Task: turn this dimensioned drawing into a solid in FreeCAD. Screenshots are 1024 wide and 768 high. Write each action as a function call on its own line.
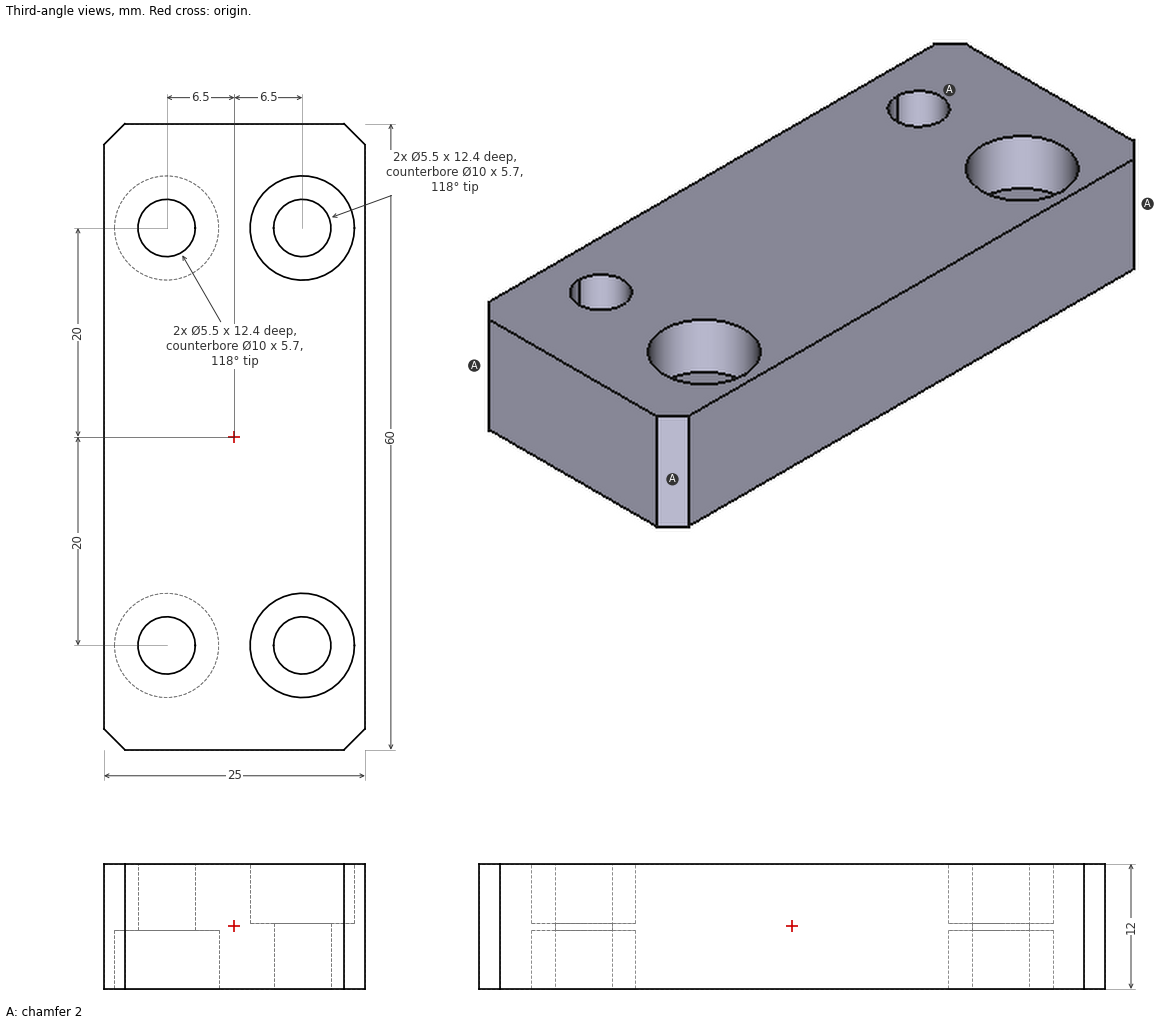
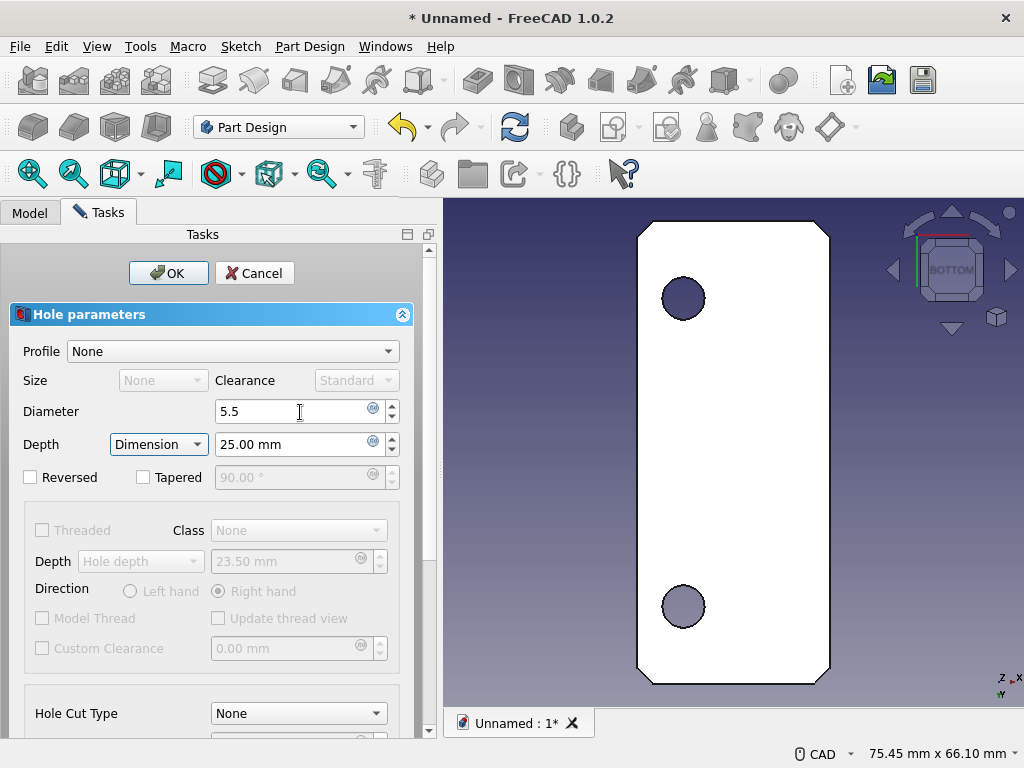
triple_click(300, 444)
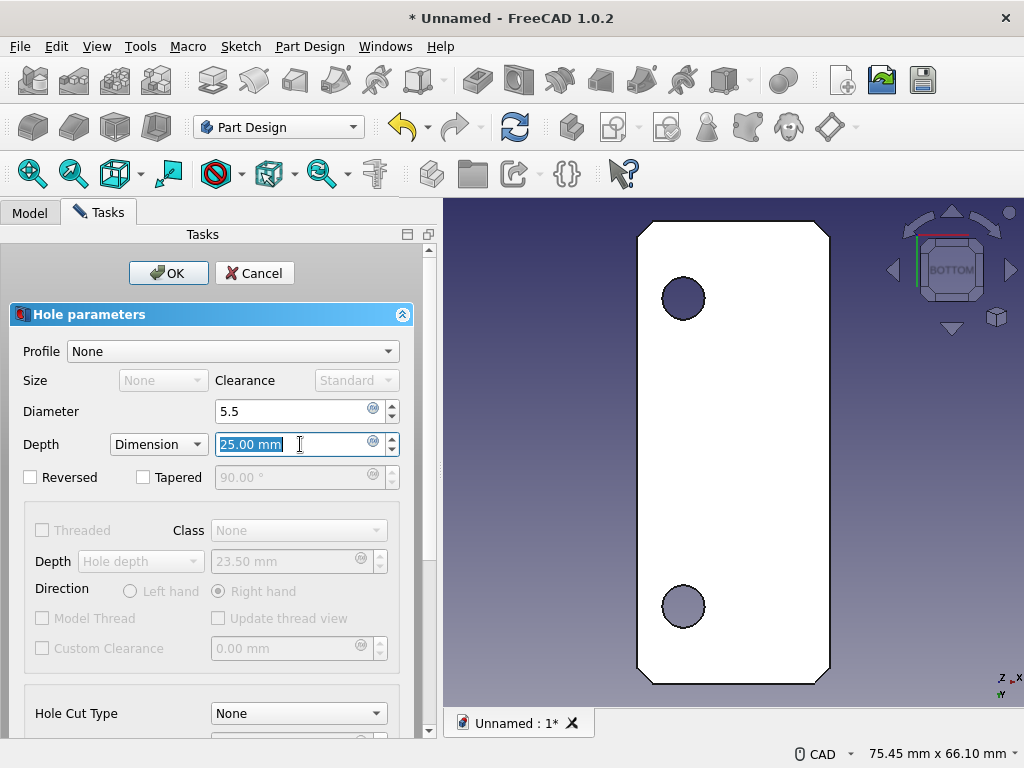
text(12.4)
key(Tab)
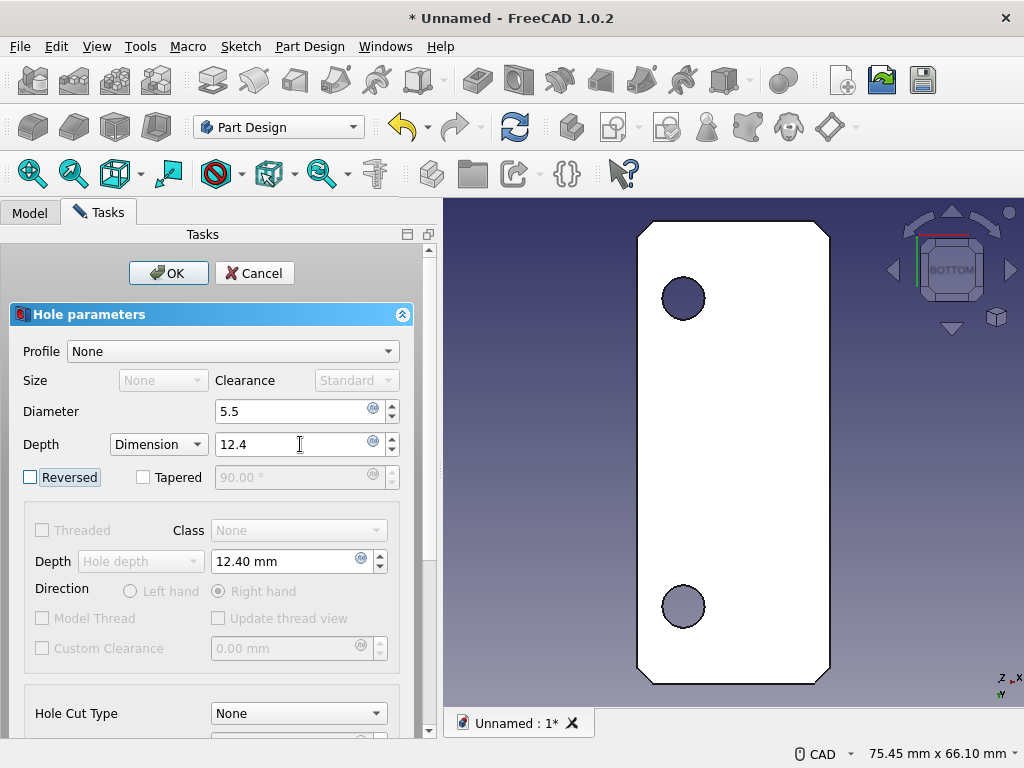
click(300, 714)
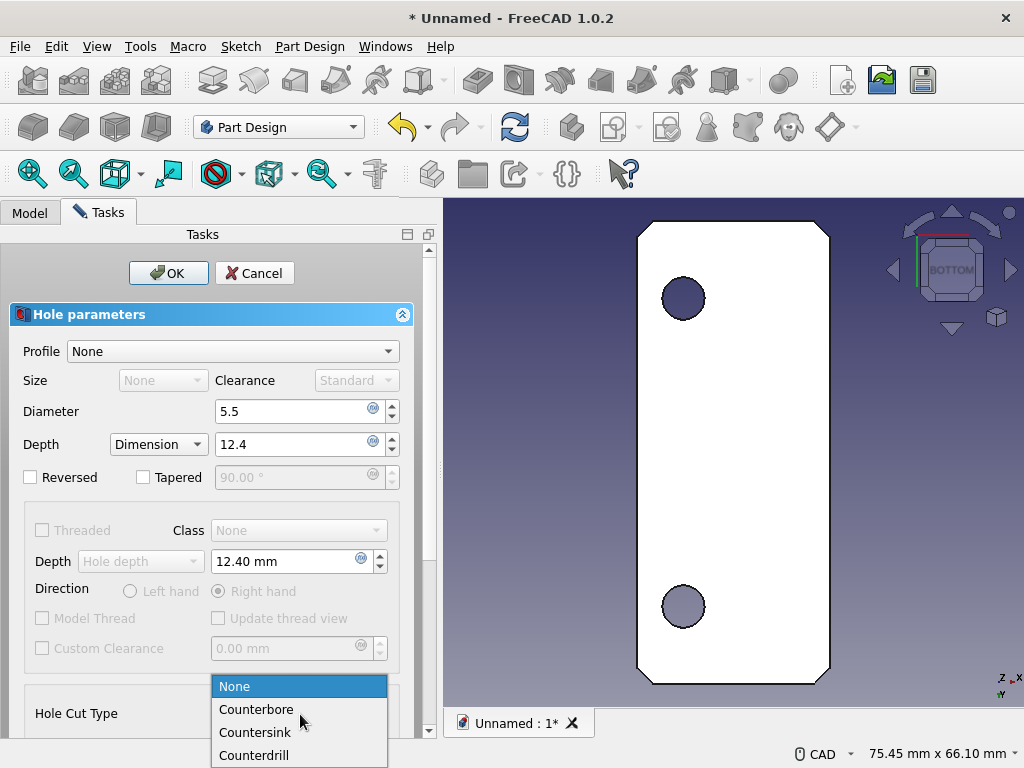
click(298, 710)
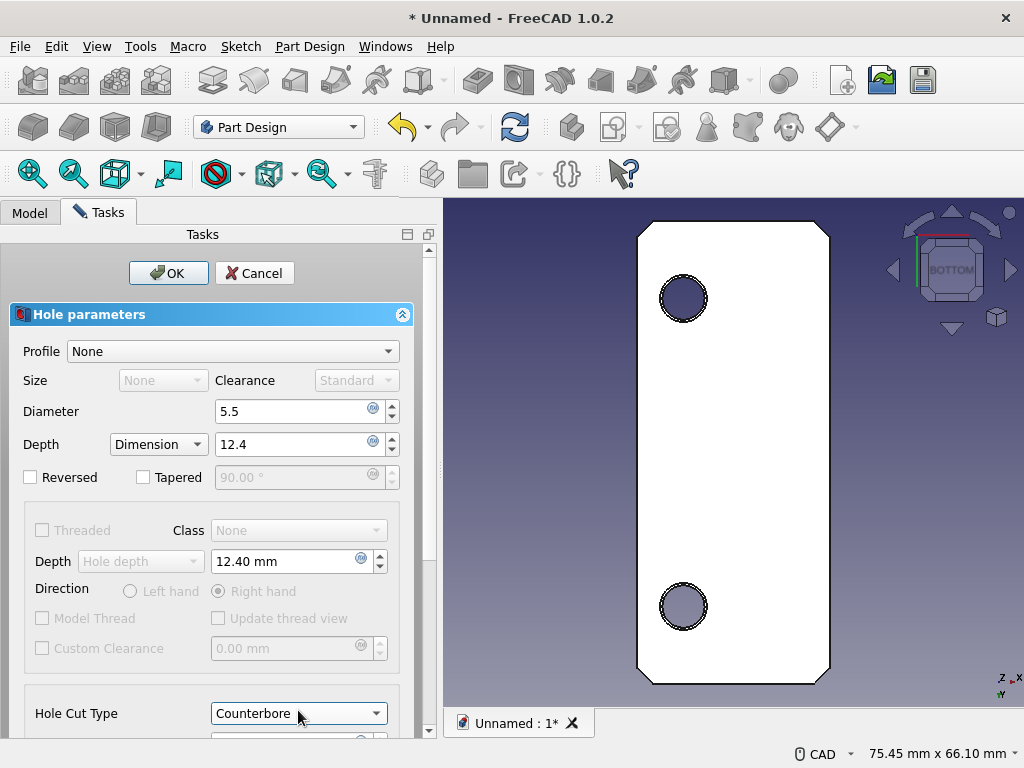
scroll(429, 491, down, 2)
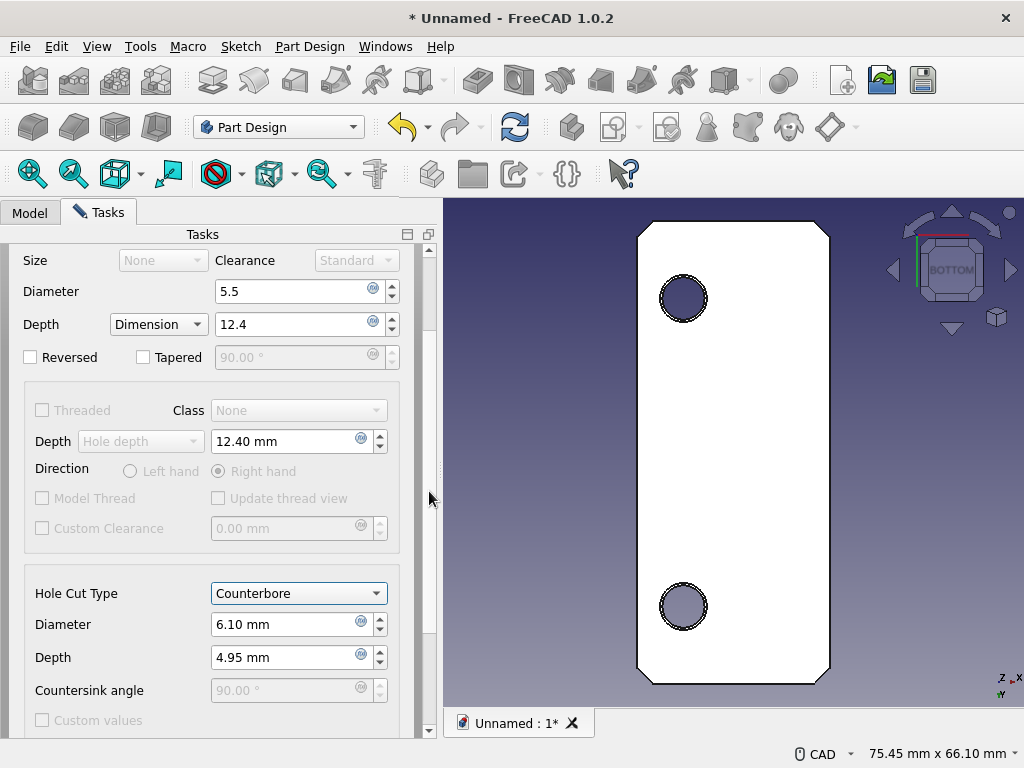
triple_click(292, 624)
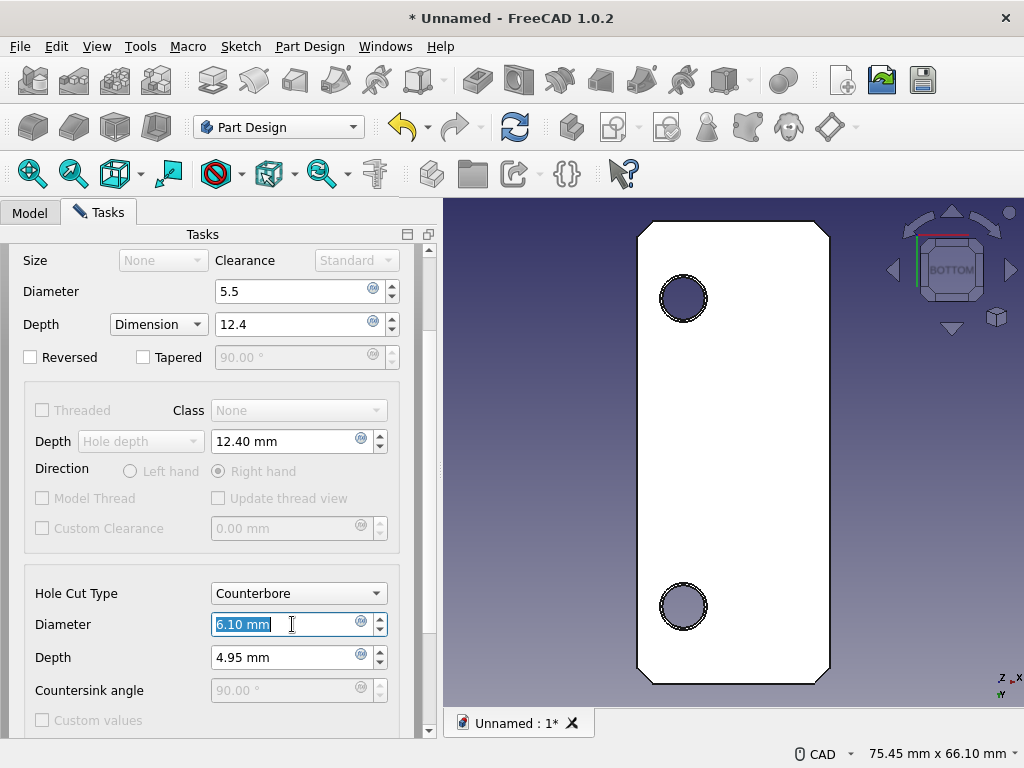
text(10)
key(Tab)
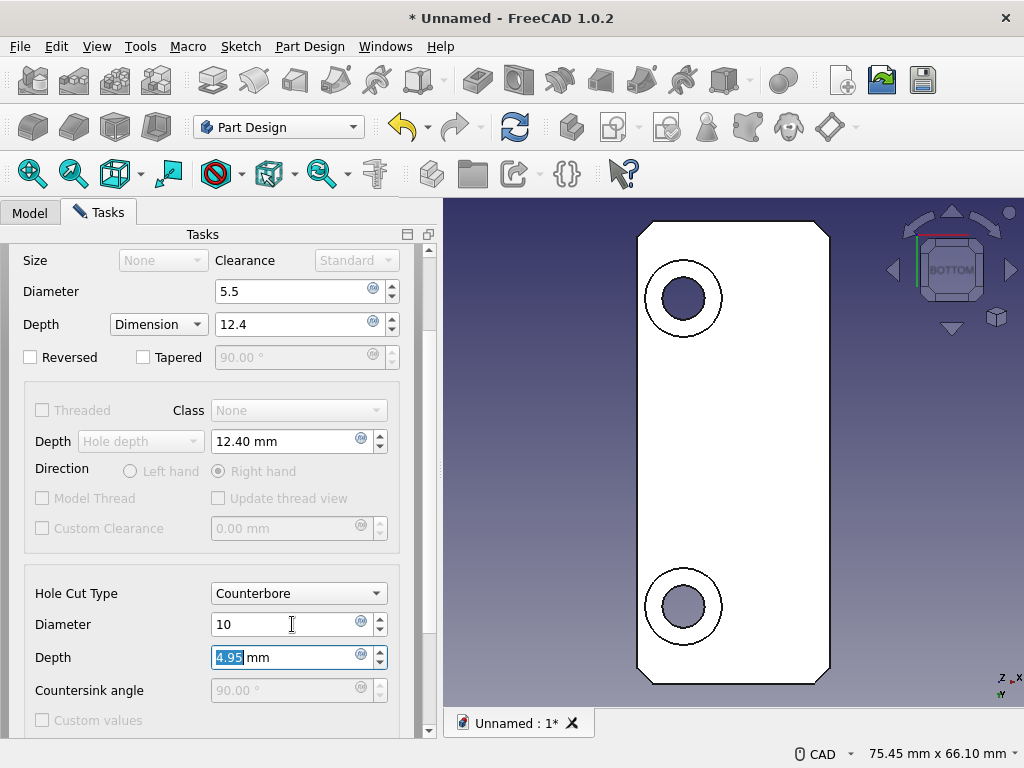
text(5.7)
key(Tab)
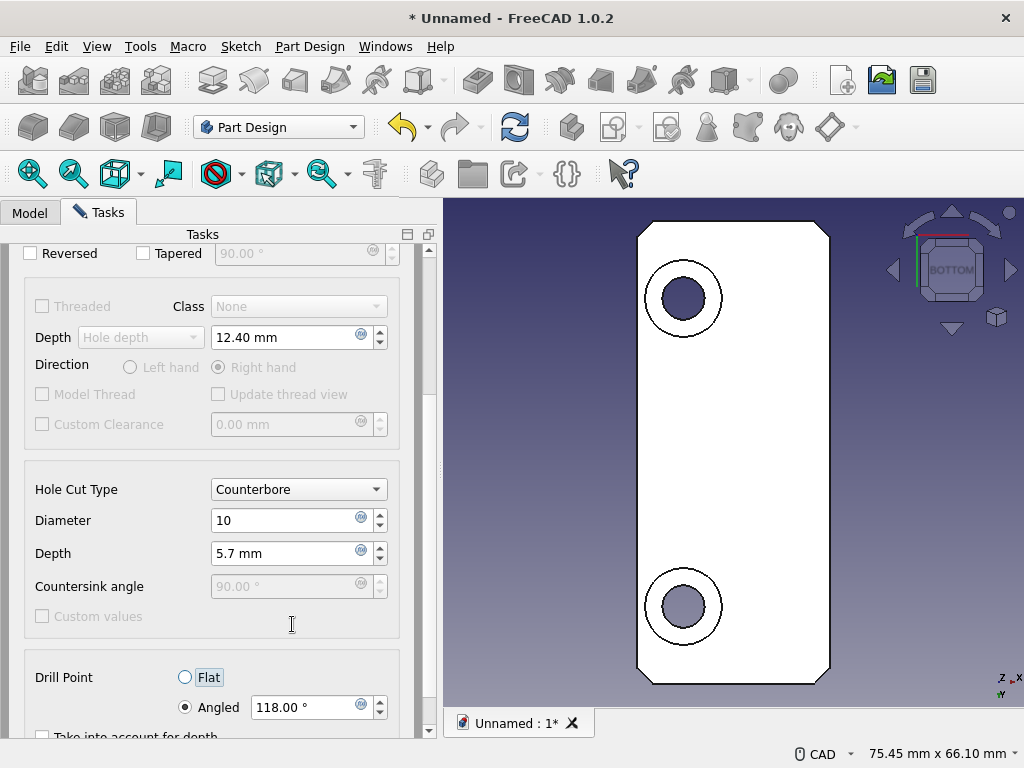
scroll(429, 491, up, 5)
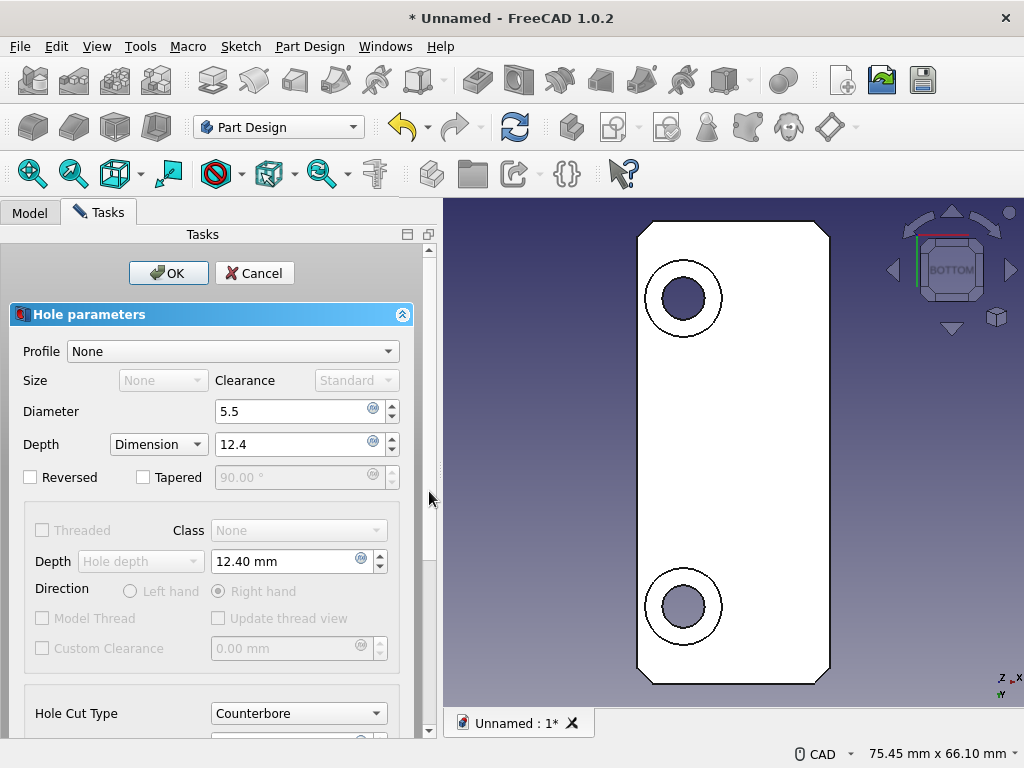
click(169, 273)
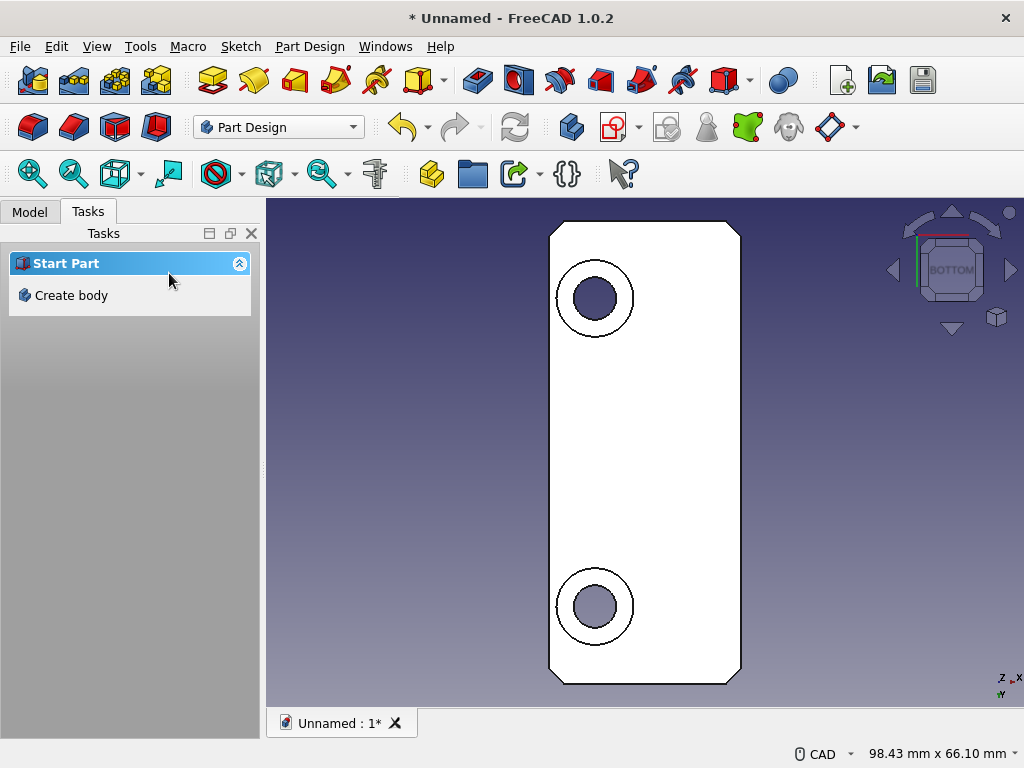
key(0)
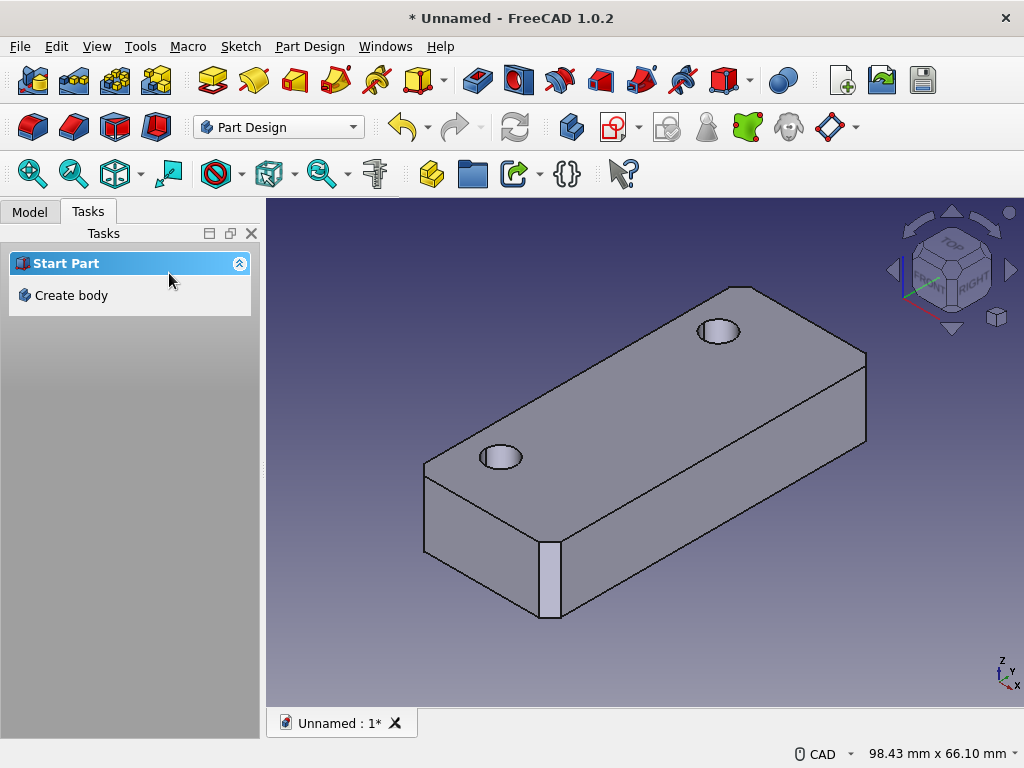
click(645, 414)